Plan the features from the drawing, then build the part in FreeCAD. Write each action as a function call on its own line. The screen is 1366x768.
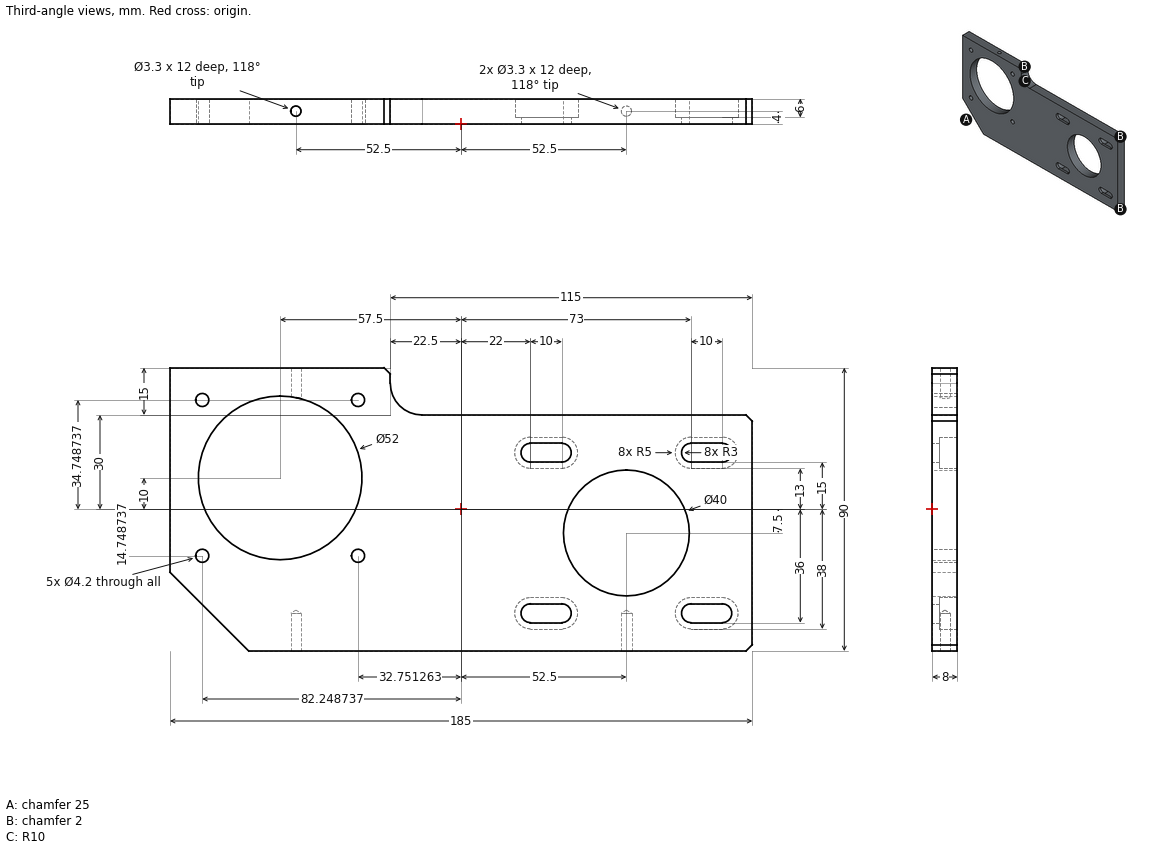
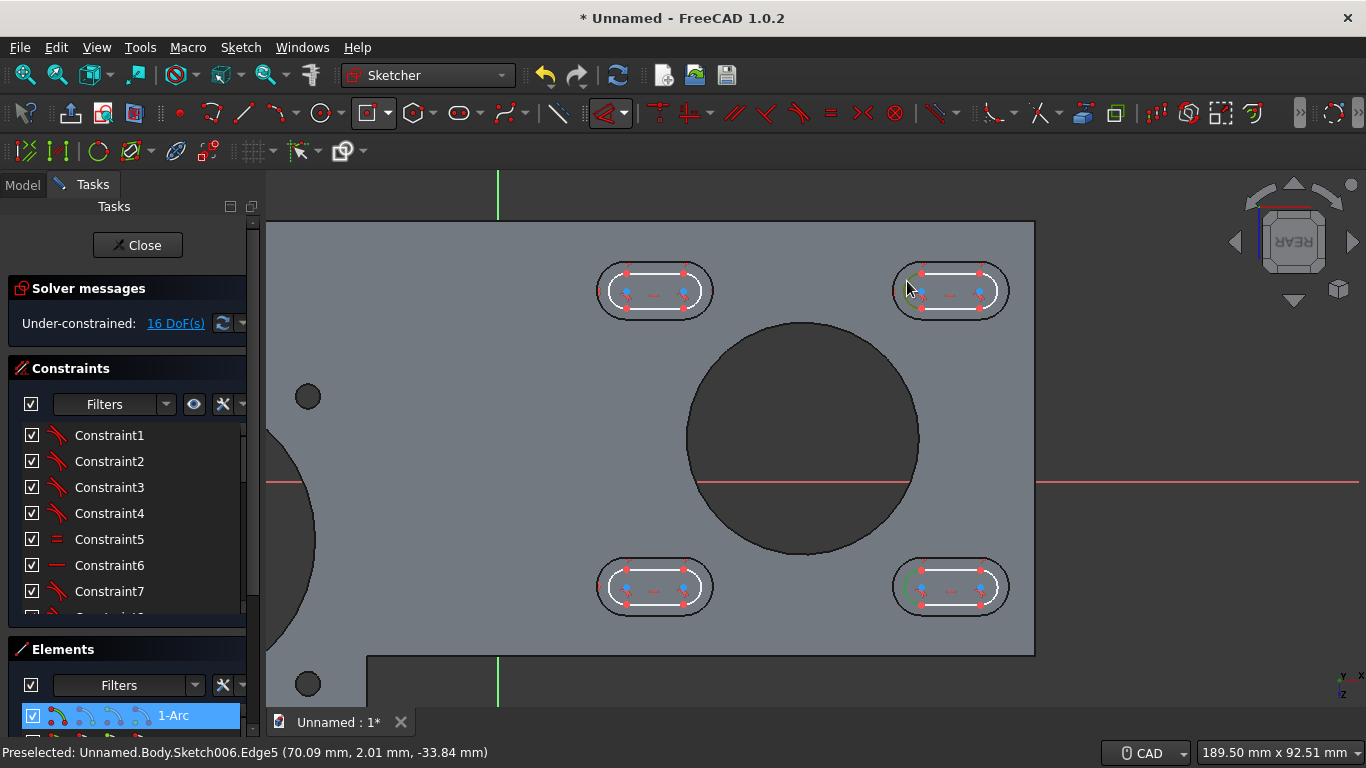
click(612, 577)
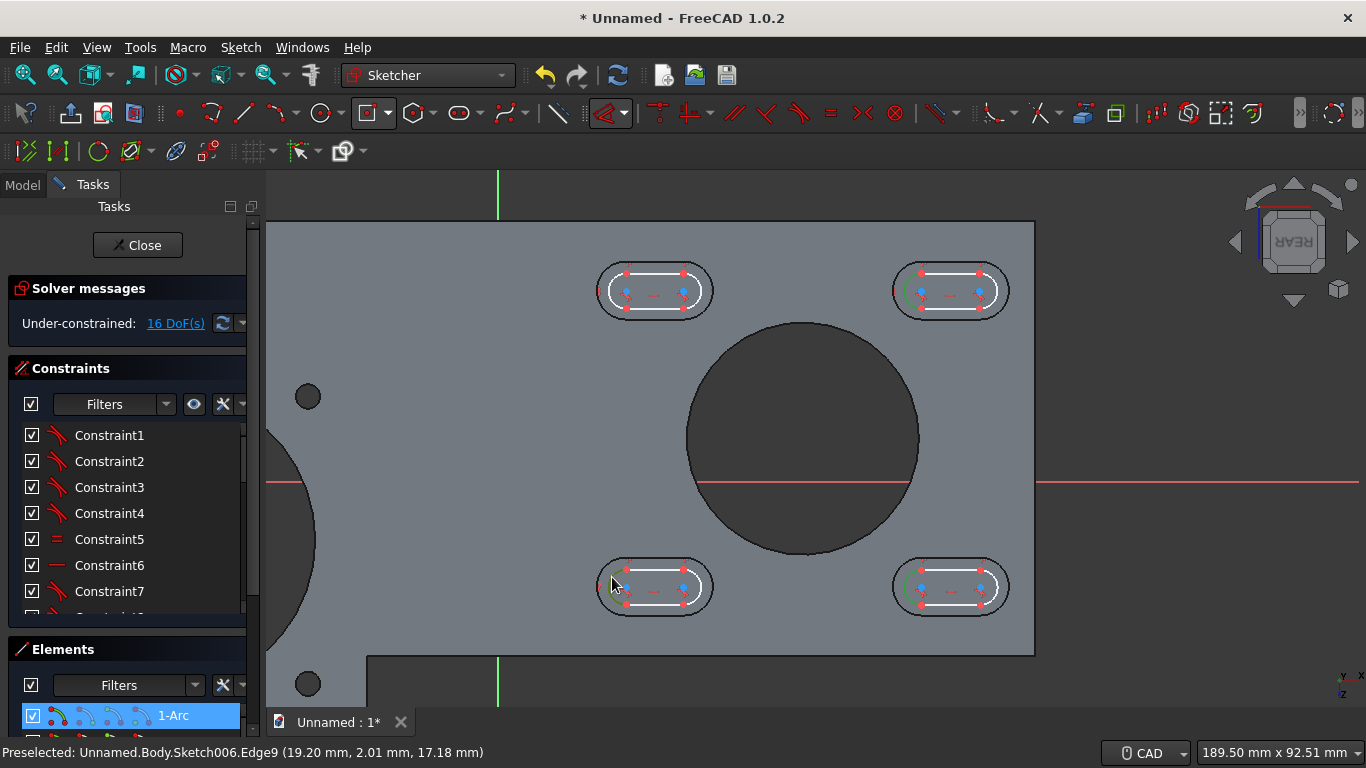
click(612, 281)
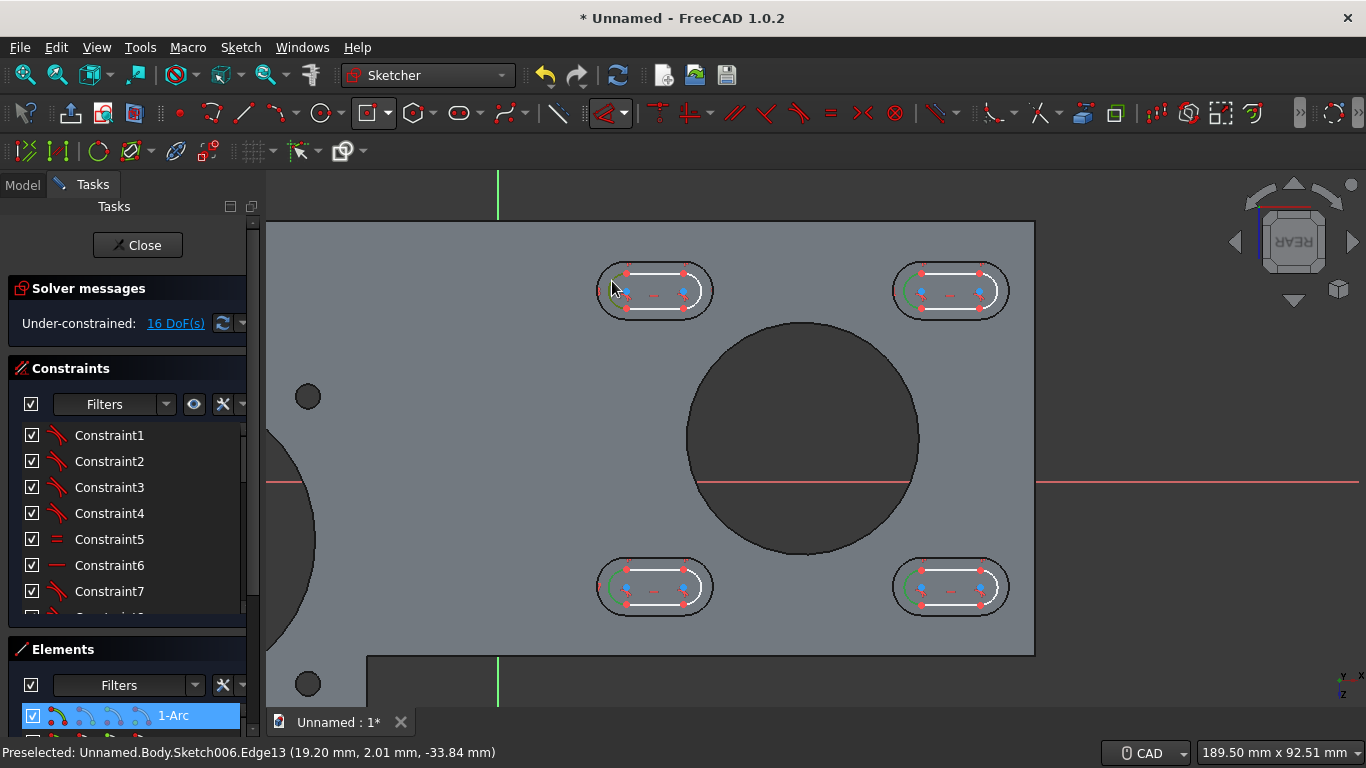
click(832, 114)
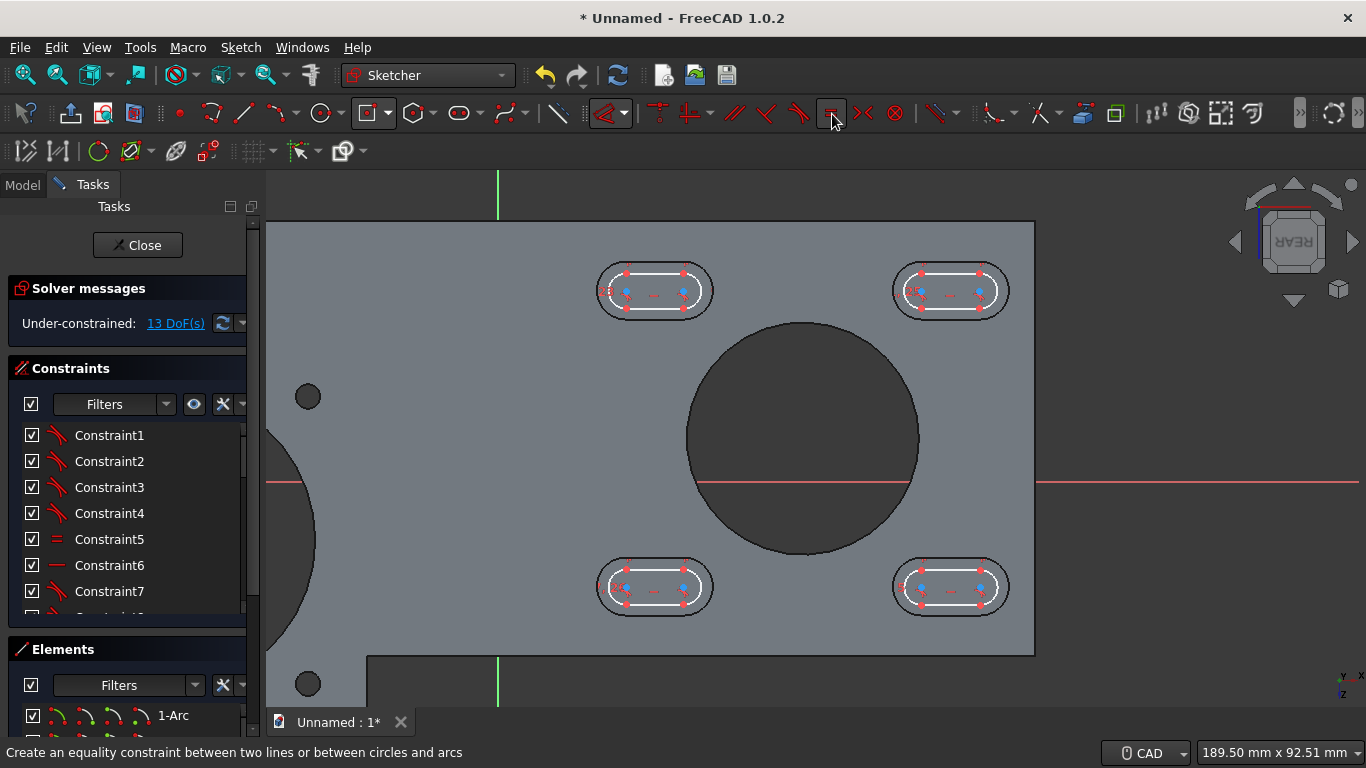
scroll(908, 577, up, 5)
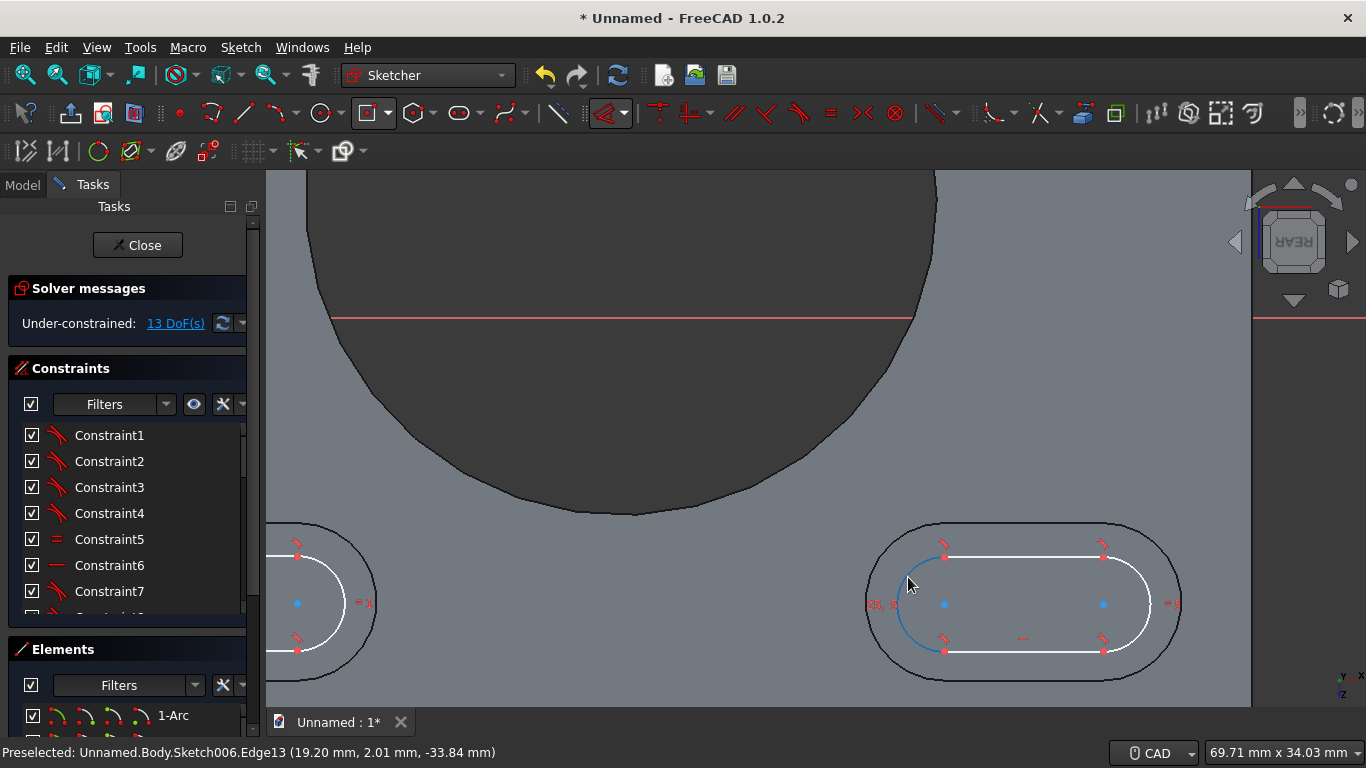
click(906, 577)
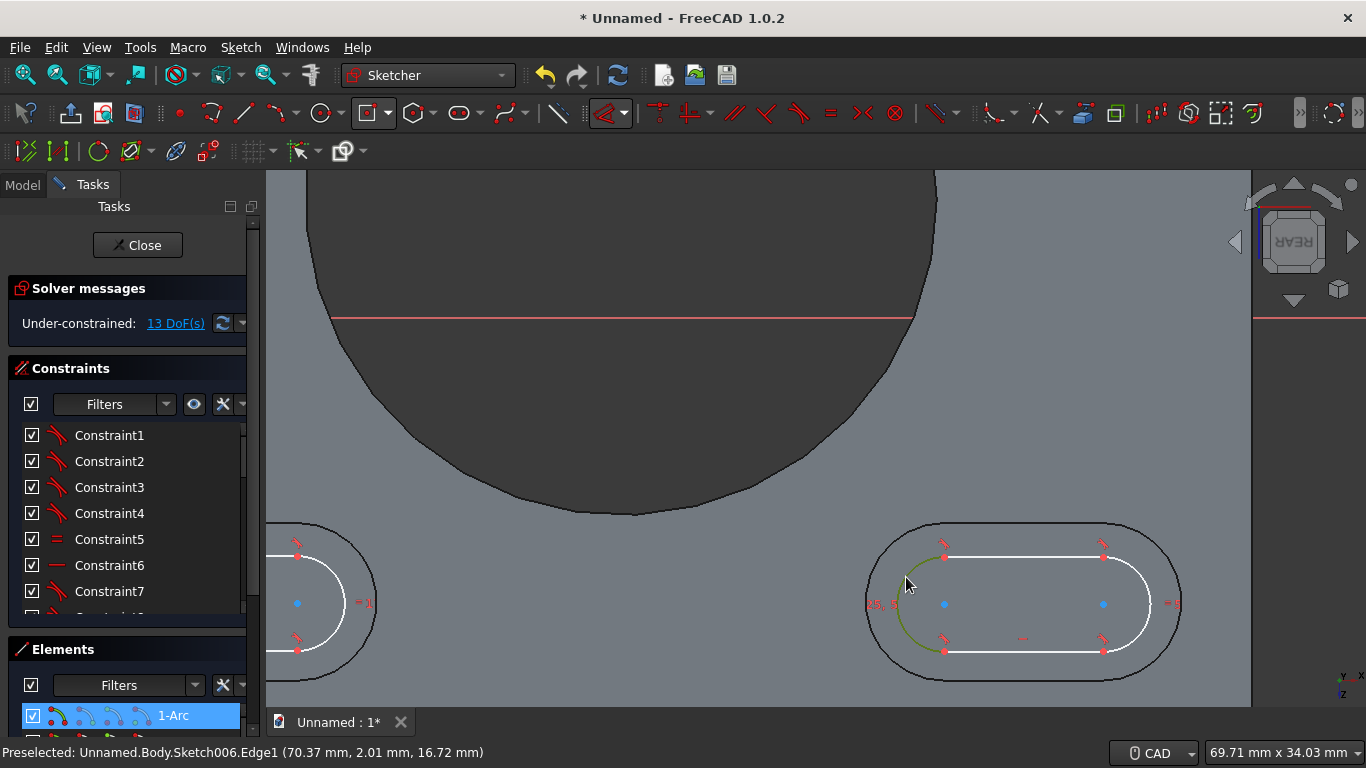
click(626, 114)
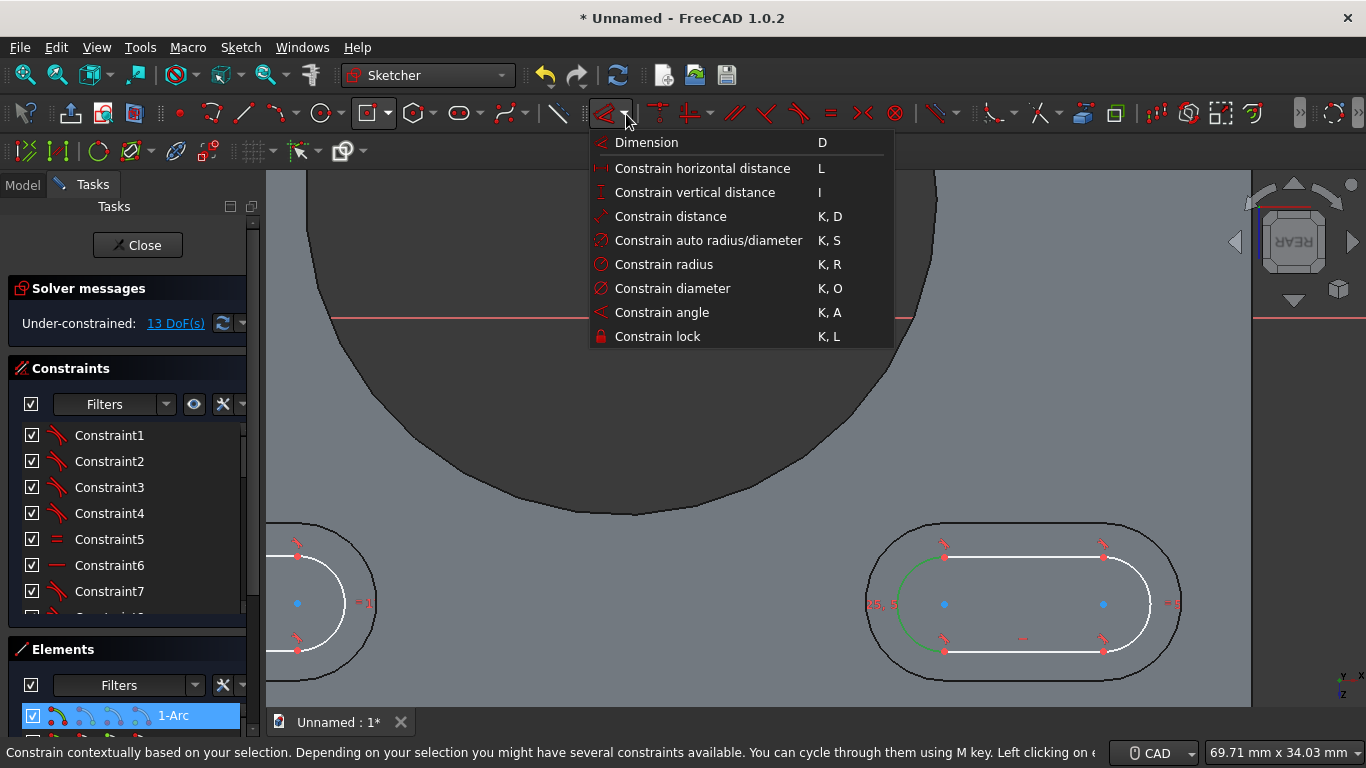
click(742, 264)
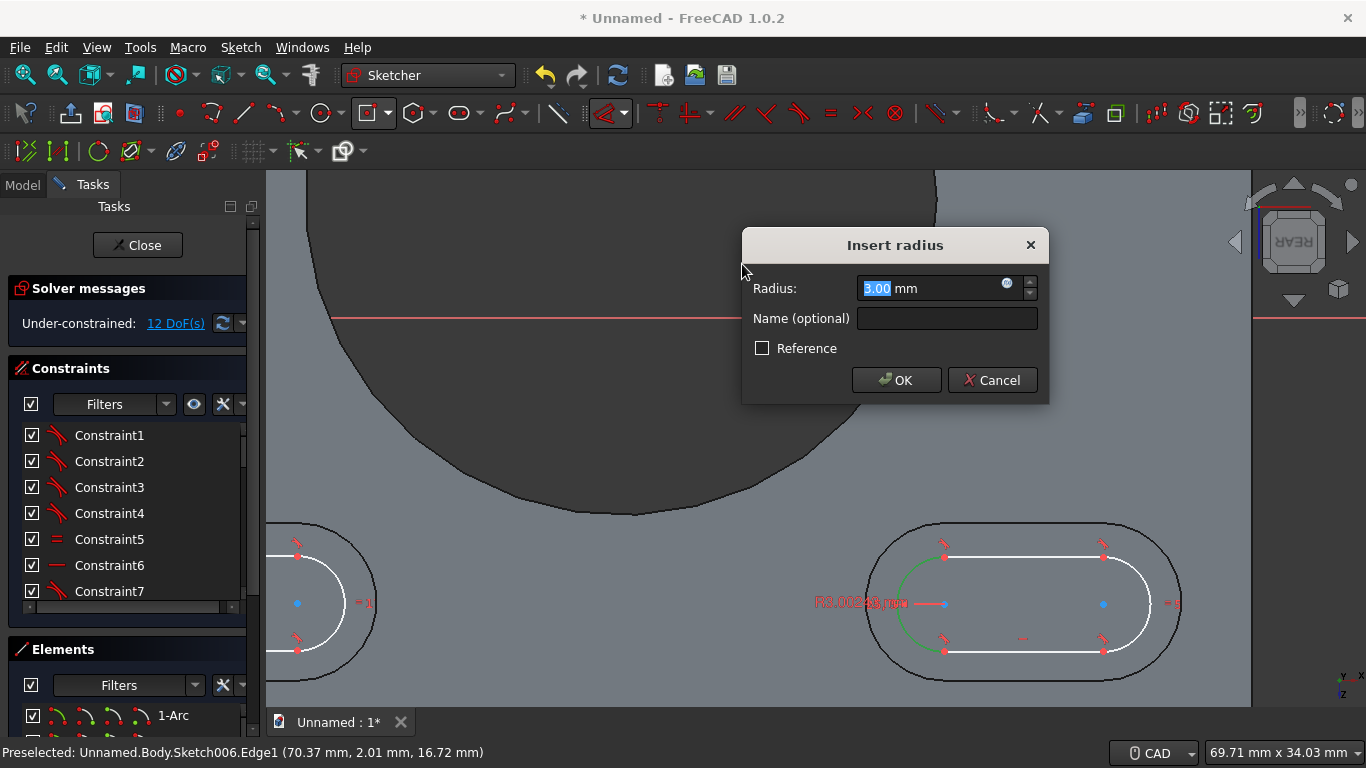
text(3)
key(Return)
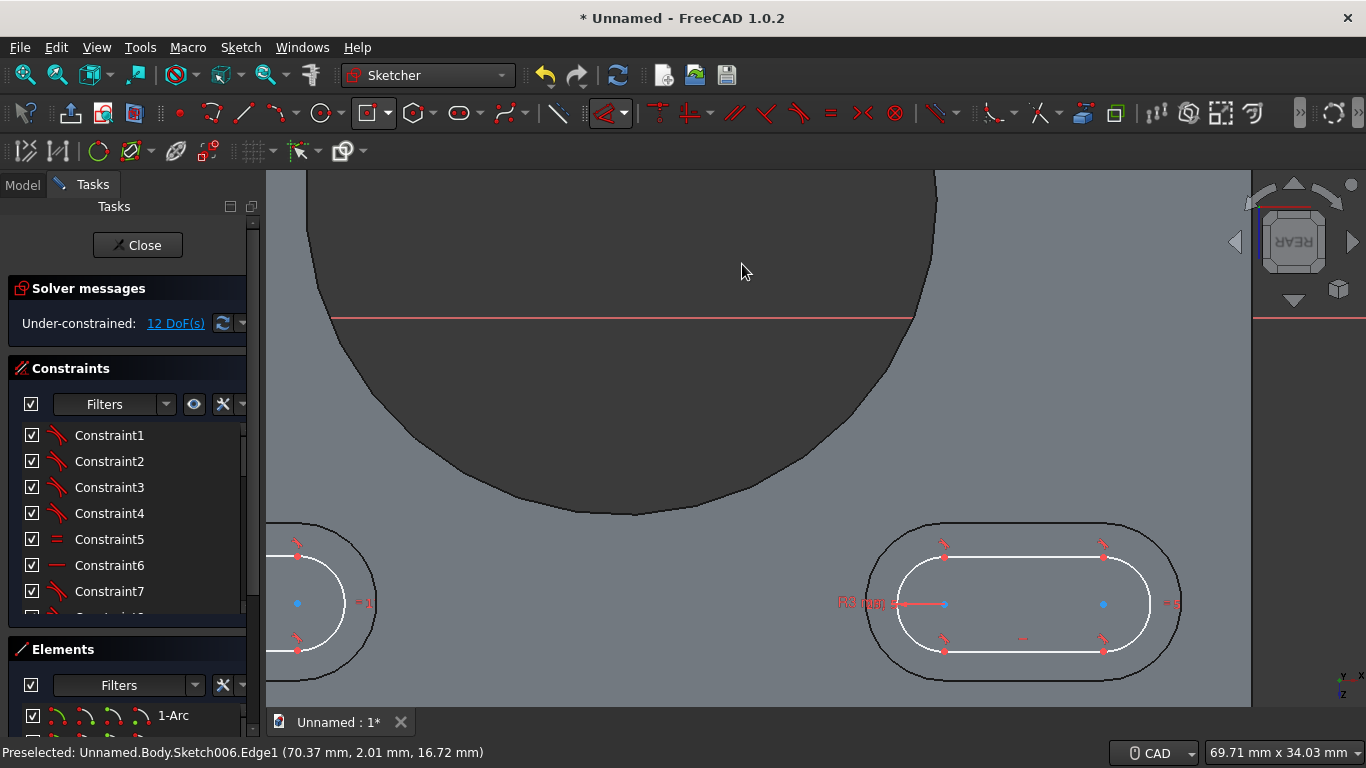
click(992, 557)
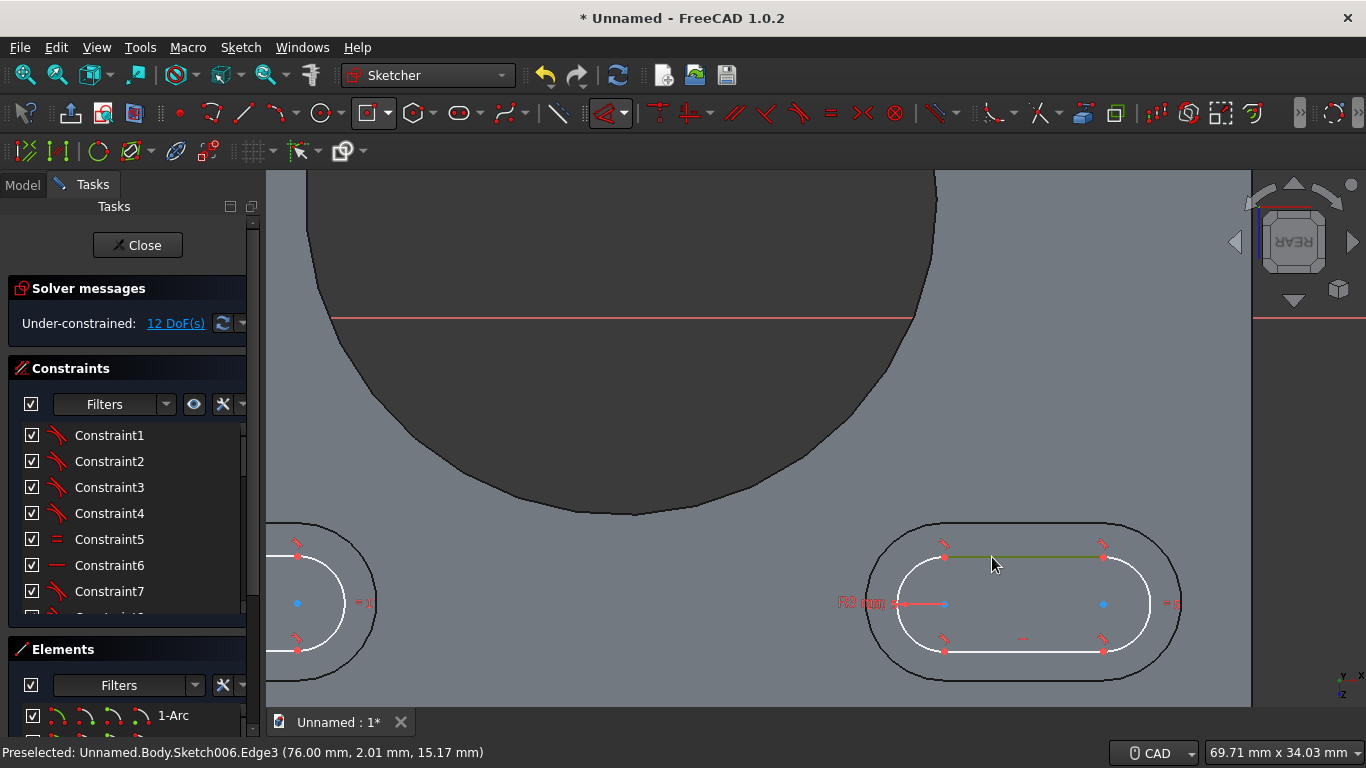
click(626, 114)